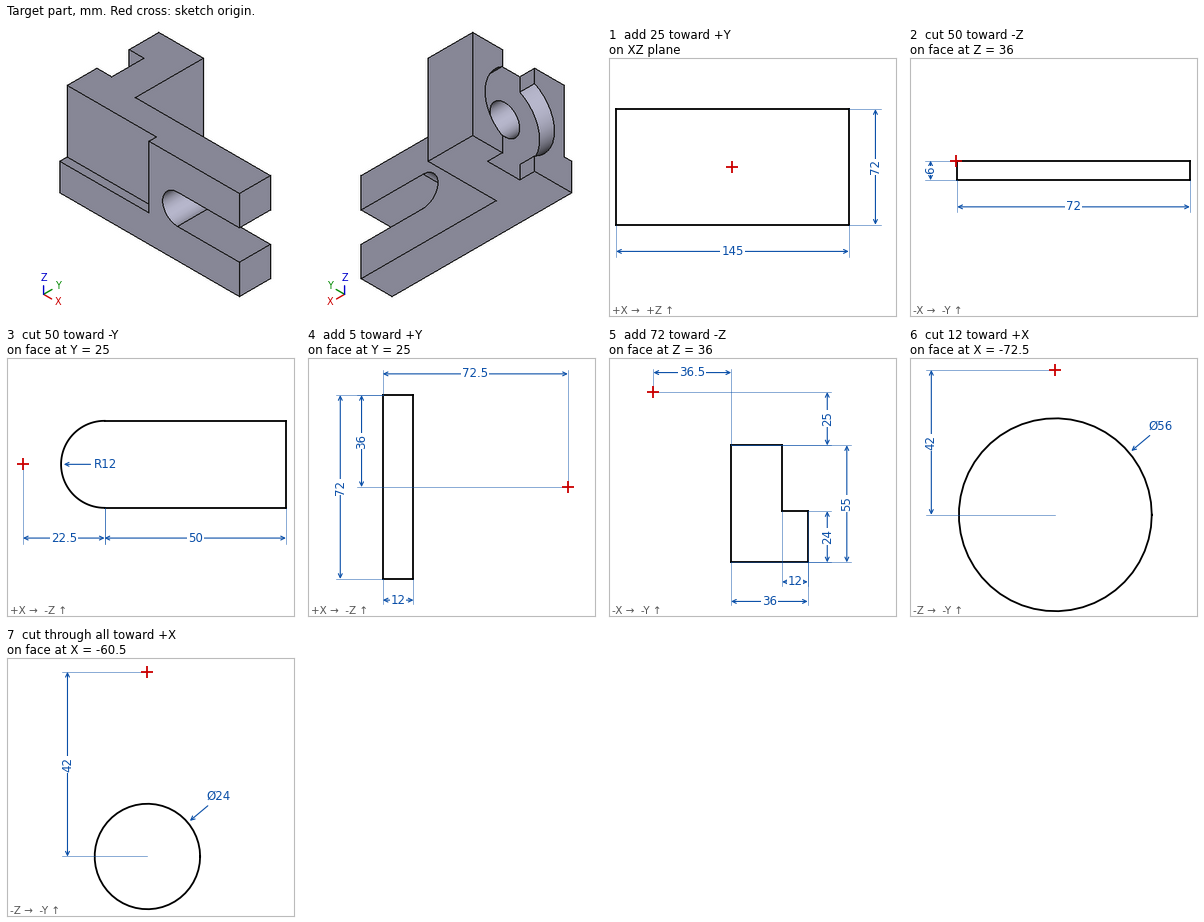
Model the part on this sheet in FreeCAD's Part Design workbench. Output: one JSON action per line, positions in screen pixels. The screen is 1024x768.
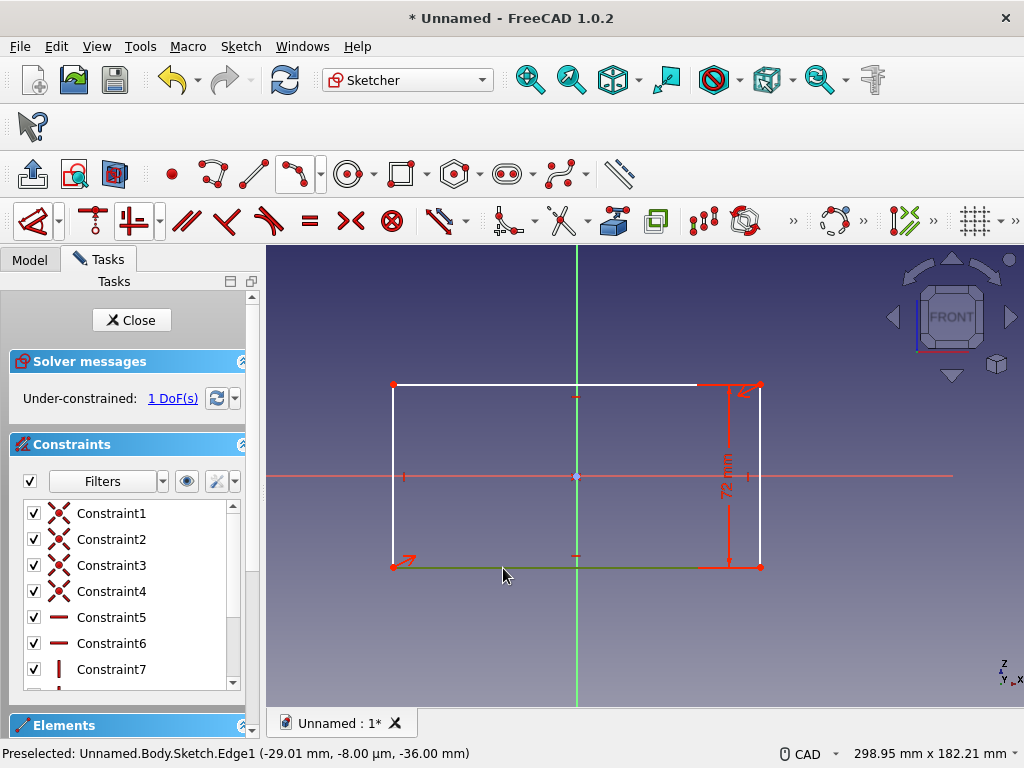
{"action": "left_click", "coordinate": [58, 222]}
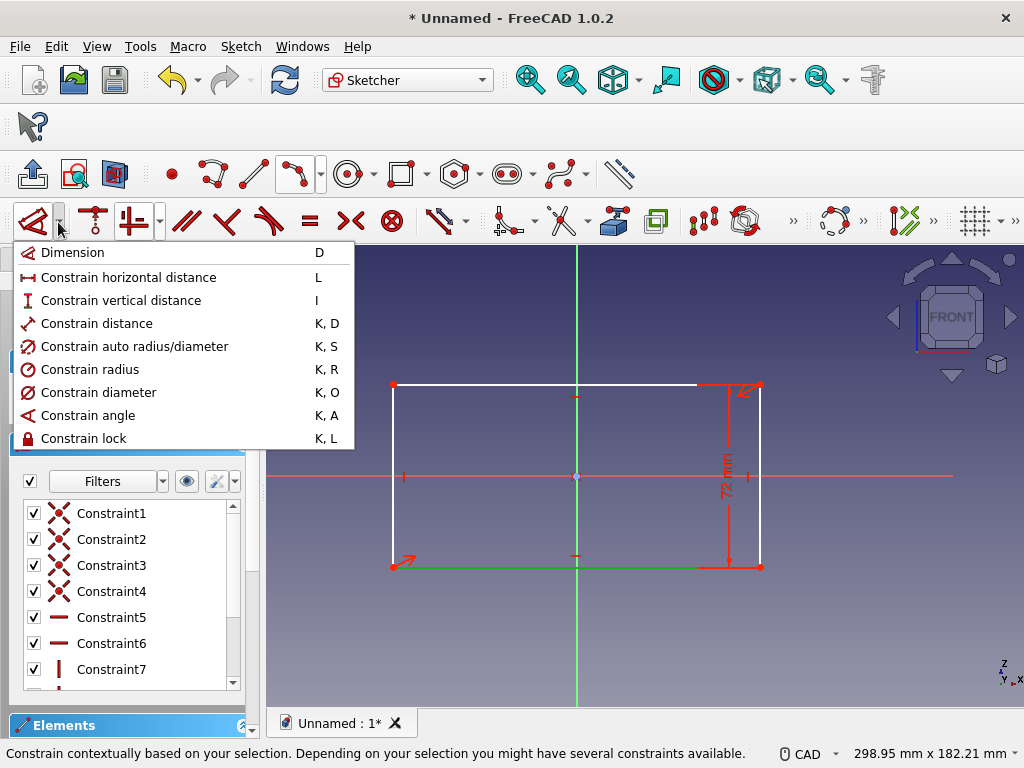
{"action": "left_click", "coordinate": [184, 278]}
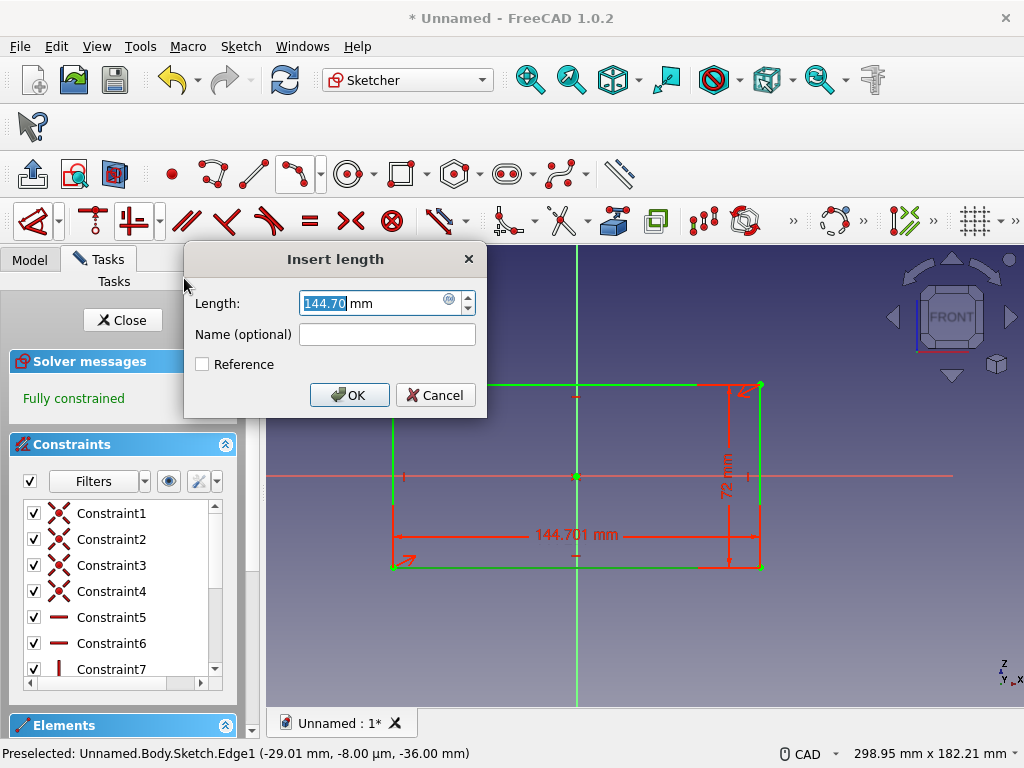
{"action": "type", "text": "145"}
{"action": "key", "text": "Return"}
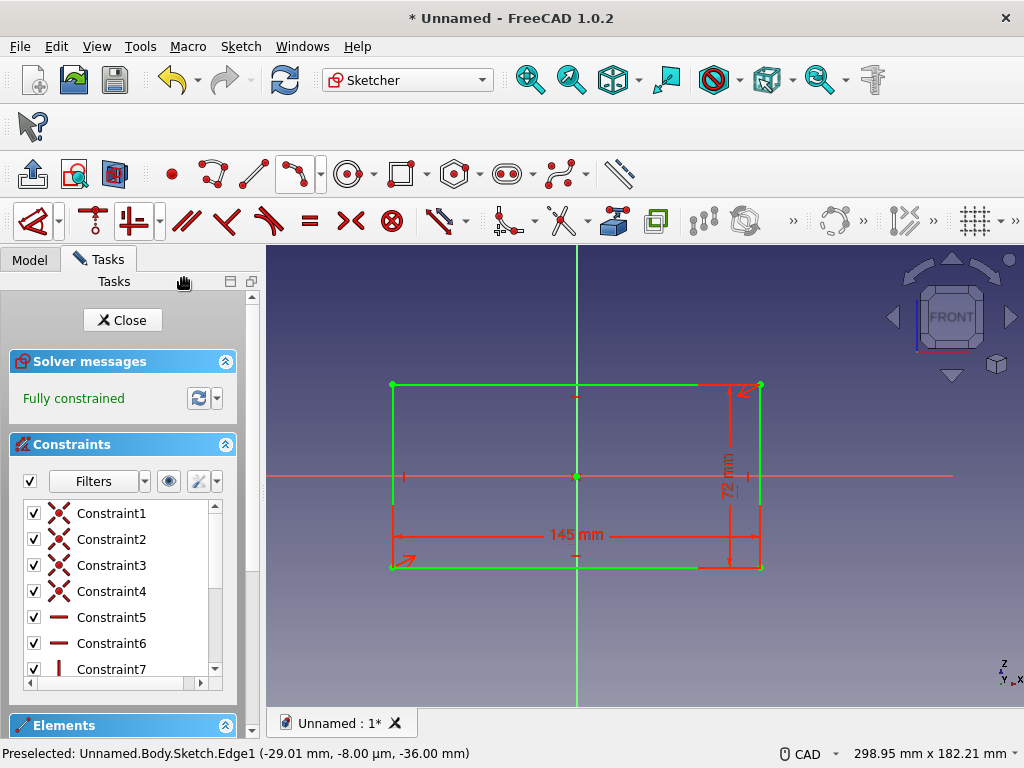
{"action": "left_click", "coordinate": [123, 320]}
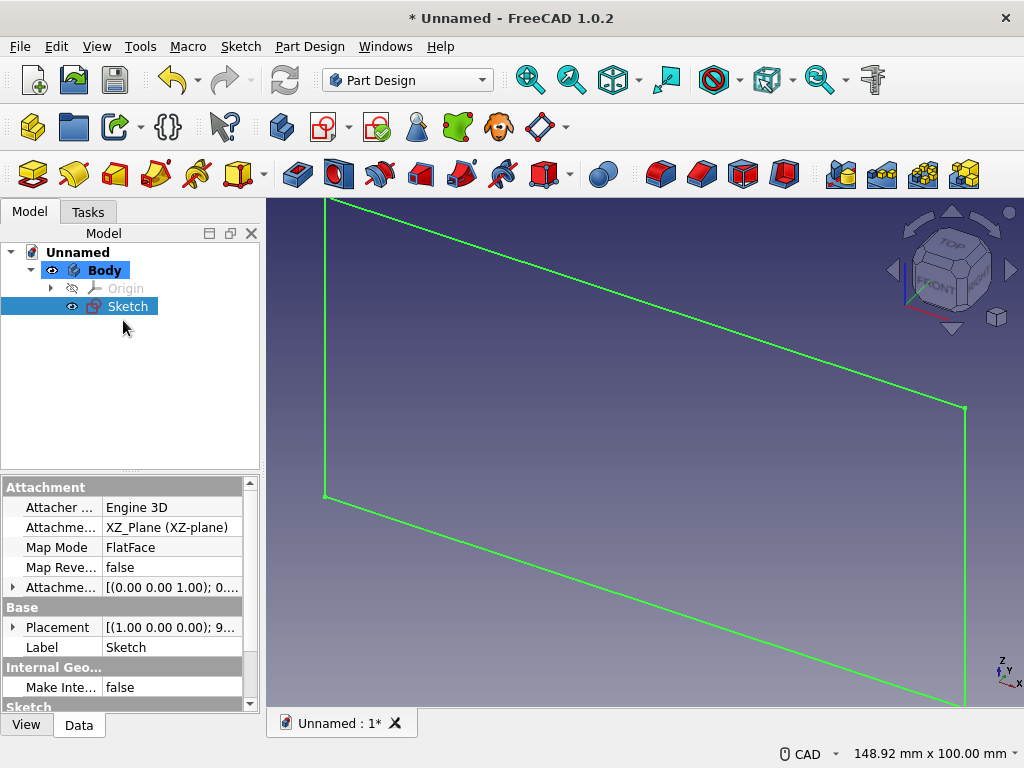
{"action": "left_click", "coordinate": [33, 174]}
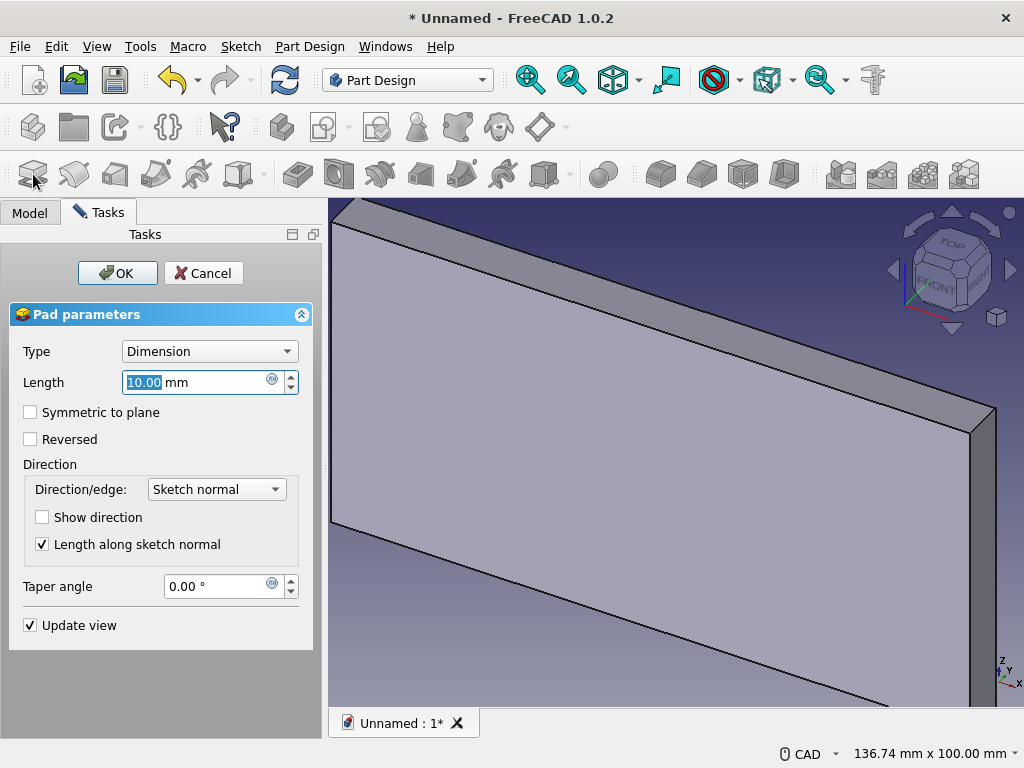
{"action": "type", "text": "25"}
{"action": "key", "text": "Tab"}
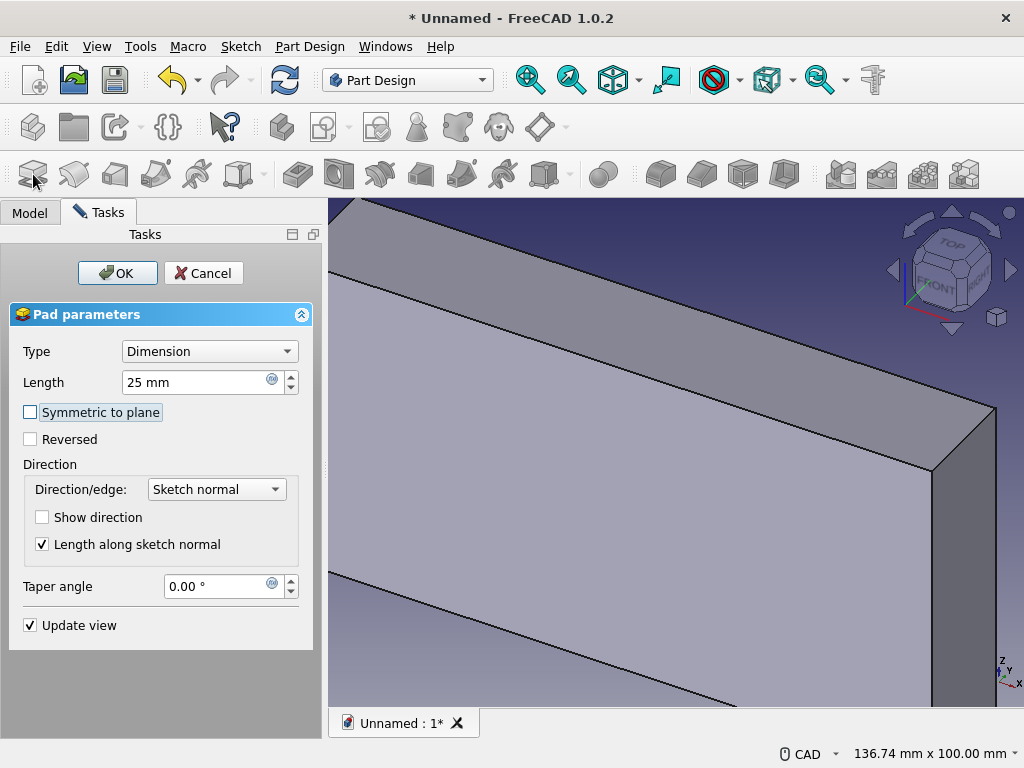
{"action": "left_click", "coordinate": [31, 439]}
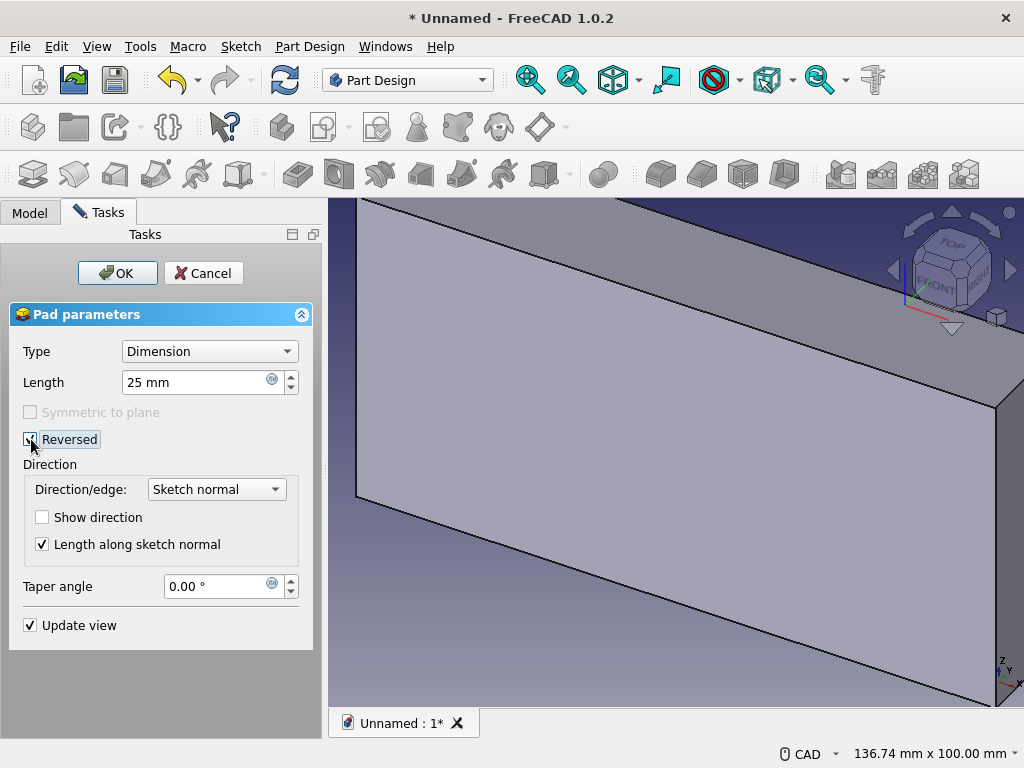
{"action": "left_click", "coordinate": [118, 273]}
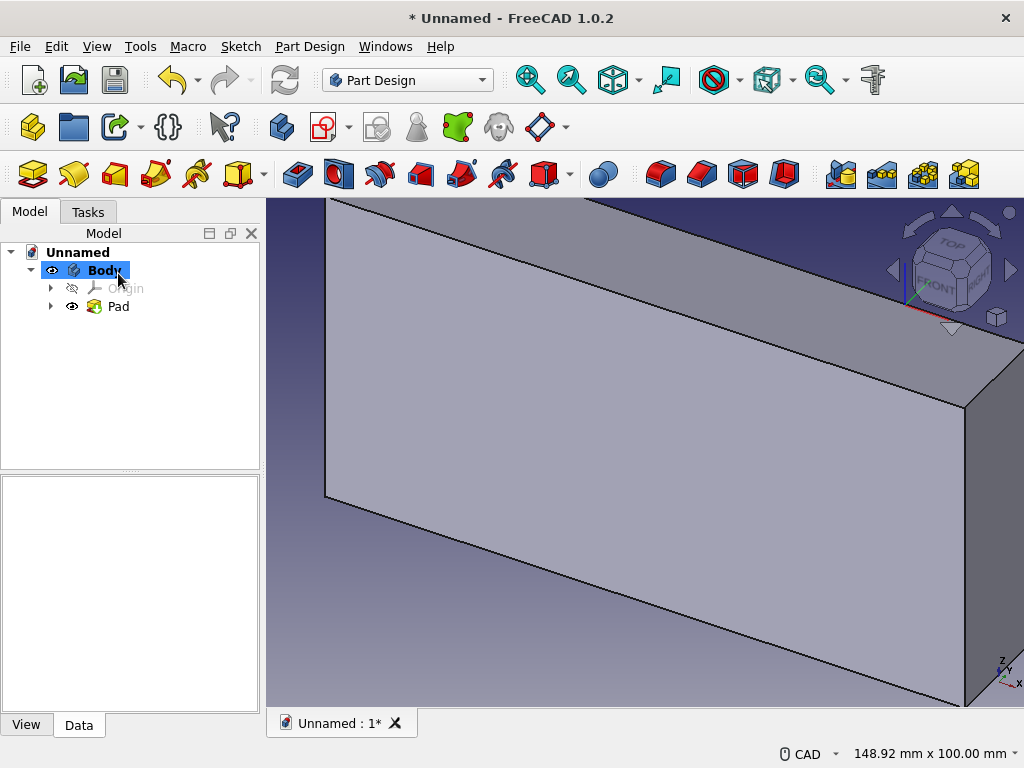
{"action": "left_click", "coordinate": [531, 80]}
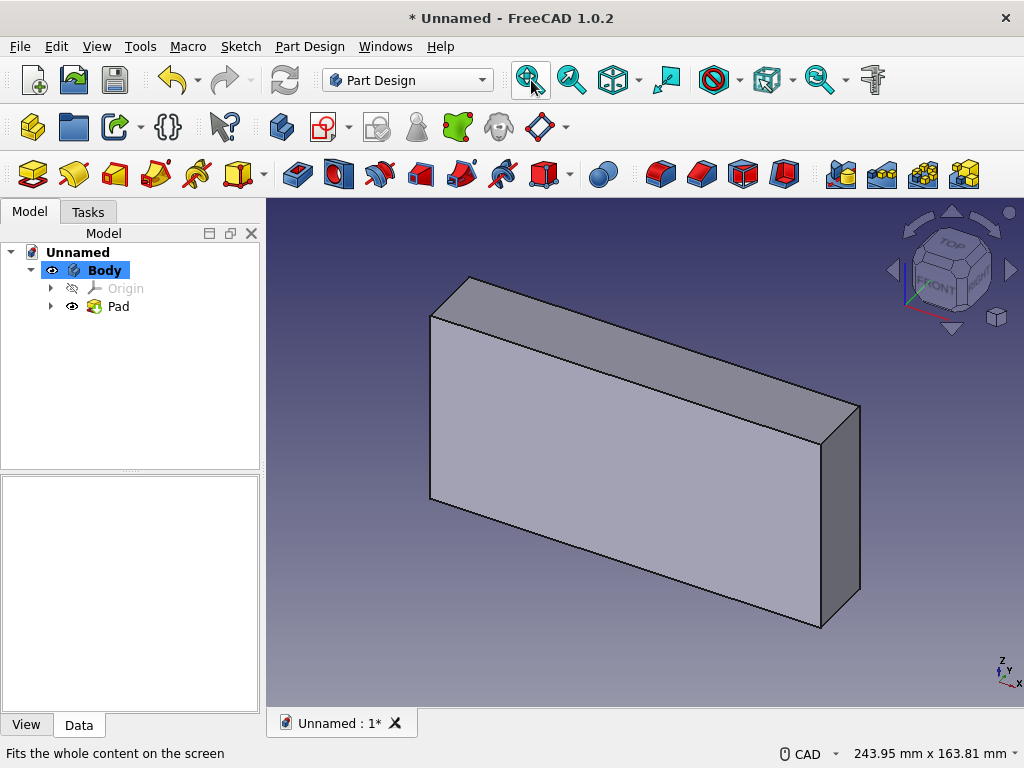
{"action": "left_click", "coordinate": [756, 397]}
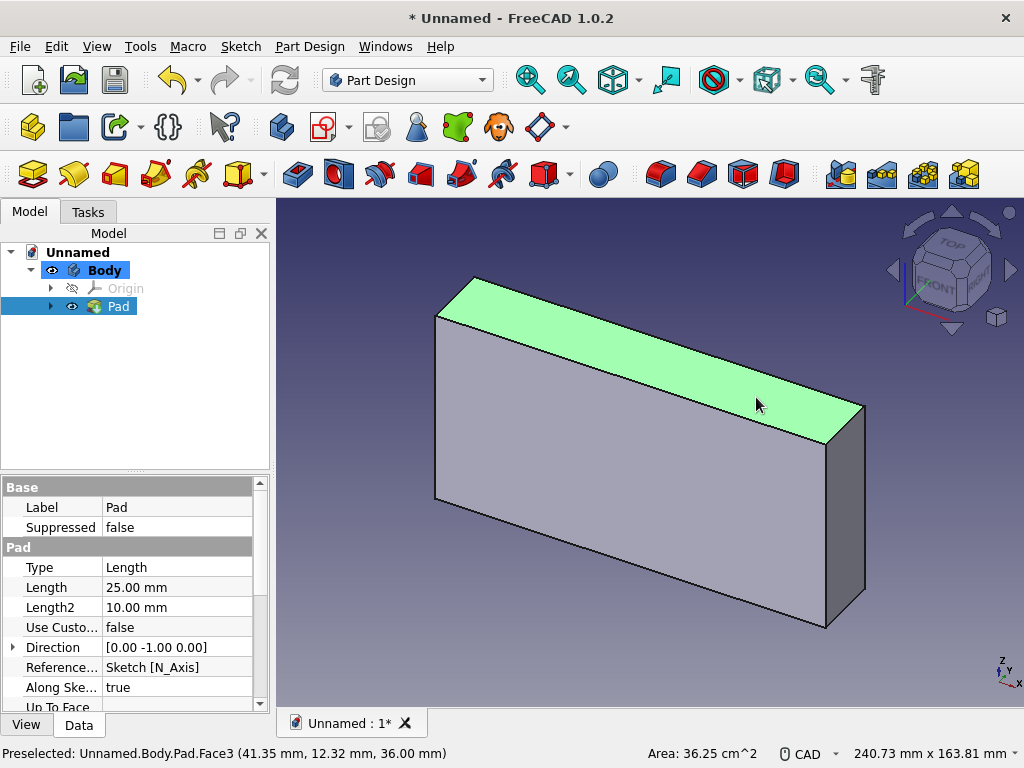
{"action": "left_click", "coordinate": [322, 128]}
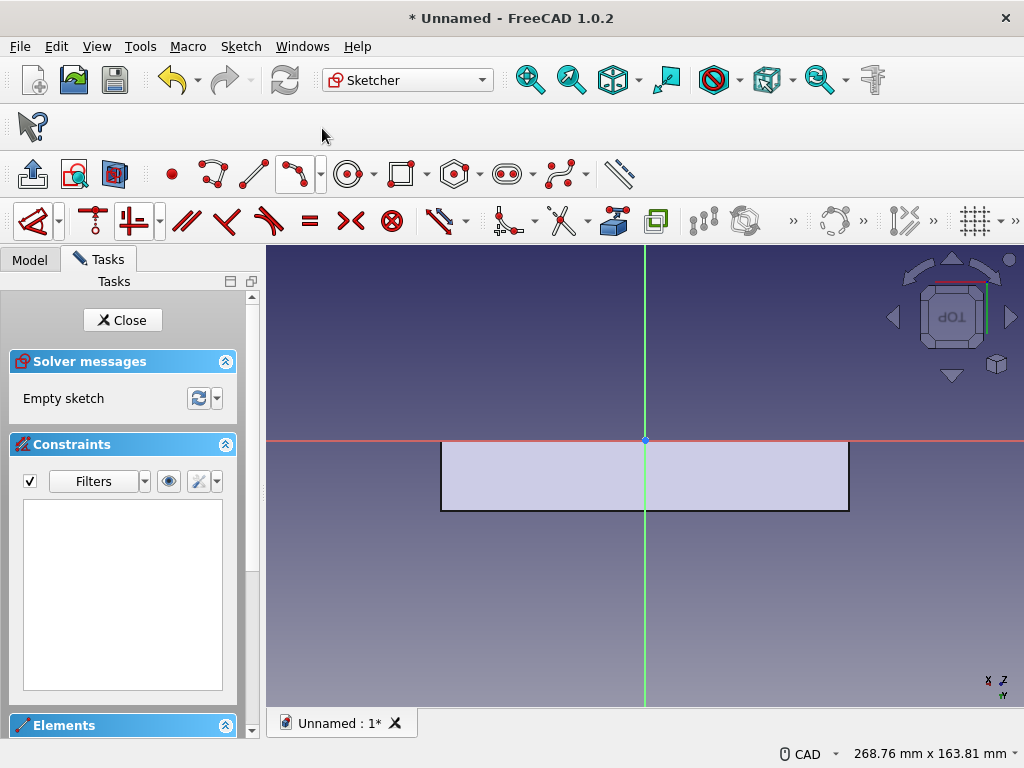
{"action": "scroll", "coordinate": [576, 476], "scroll_direction": "down", "scroll_amount": 5}